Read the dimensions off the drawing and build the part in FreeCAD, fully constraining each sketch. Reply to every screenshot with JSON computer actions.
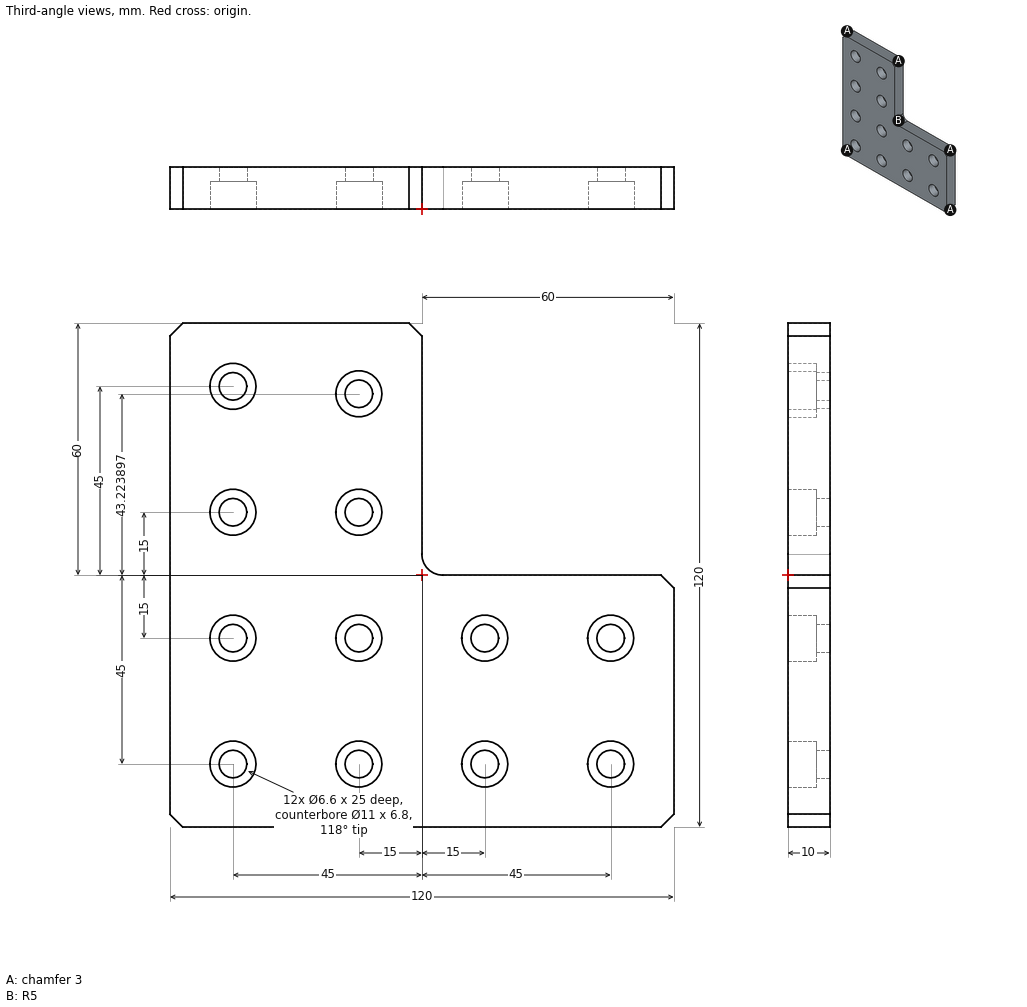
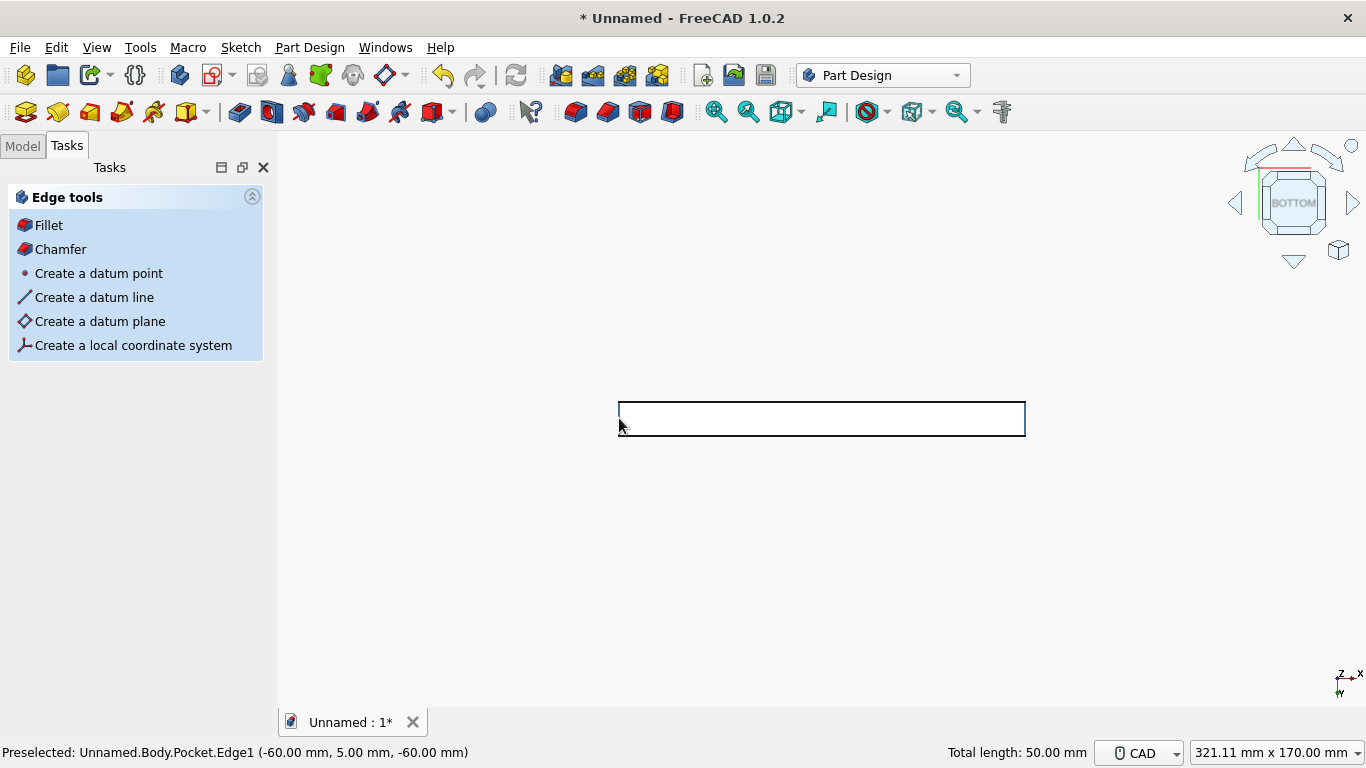
{"action": "left_click", "coordinate": [608, 112]}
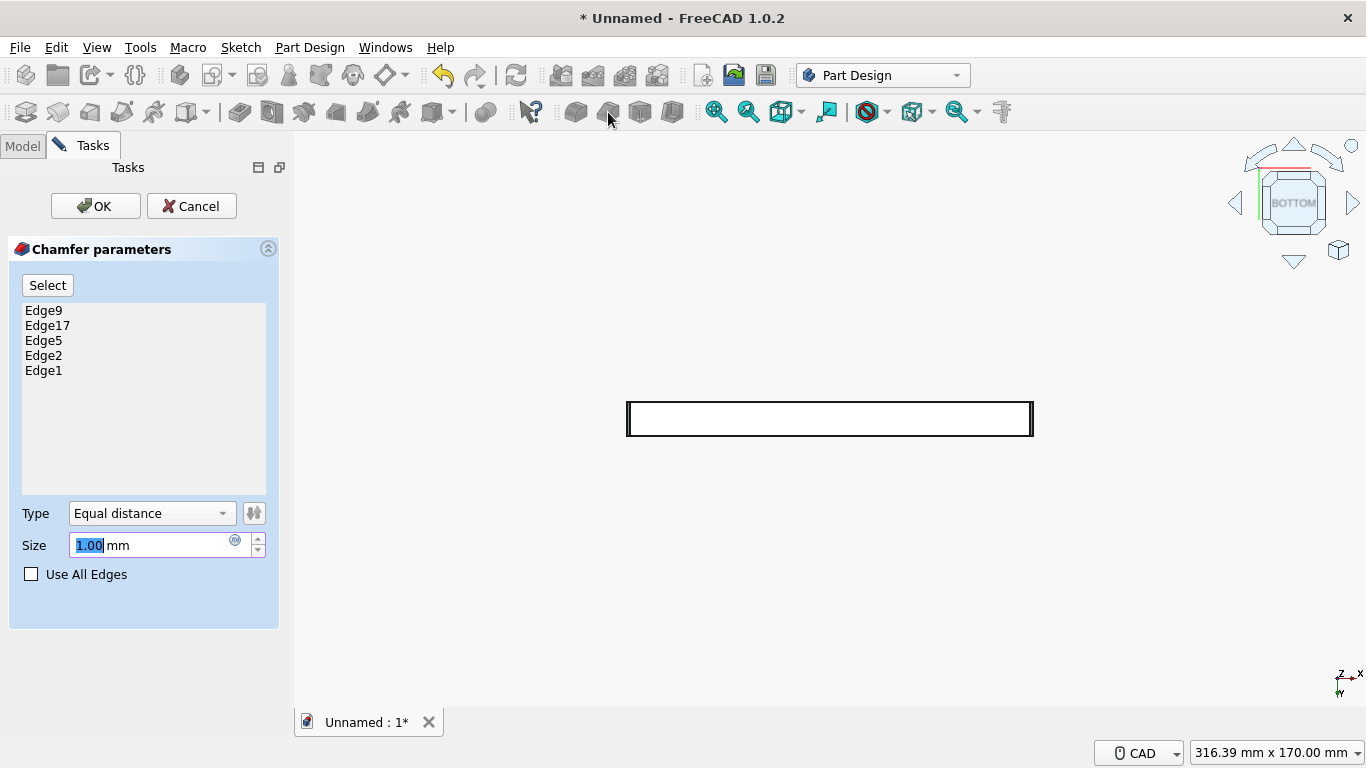
{"action": "type", "text": "3"}
{"action": "key", "text": "Tab"}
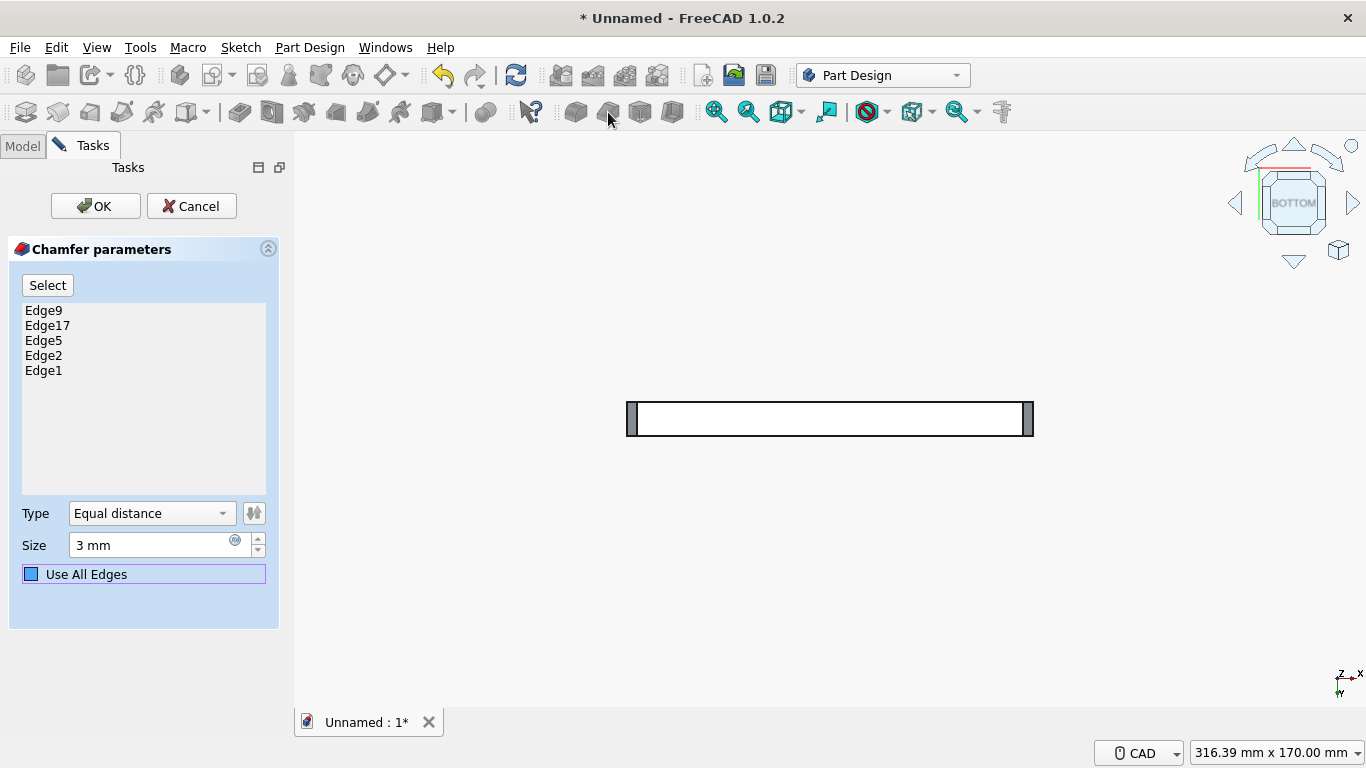
{"action": "left_click", "coordinate": [96, 206]}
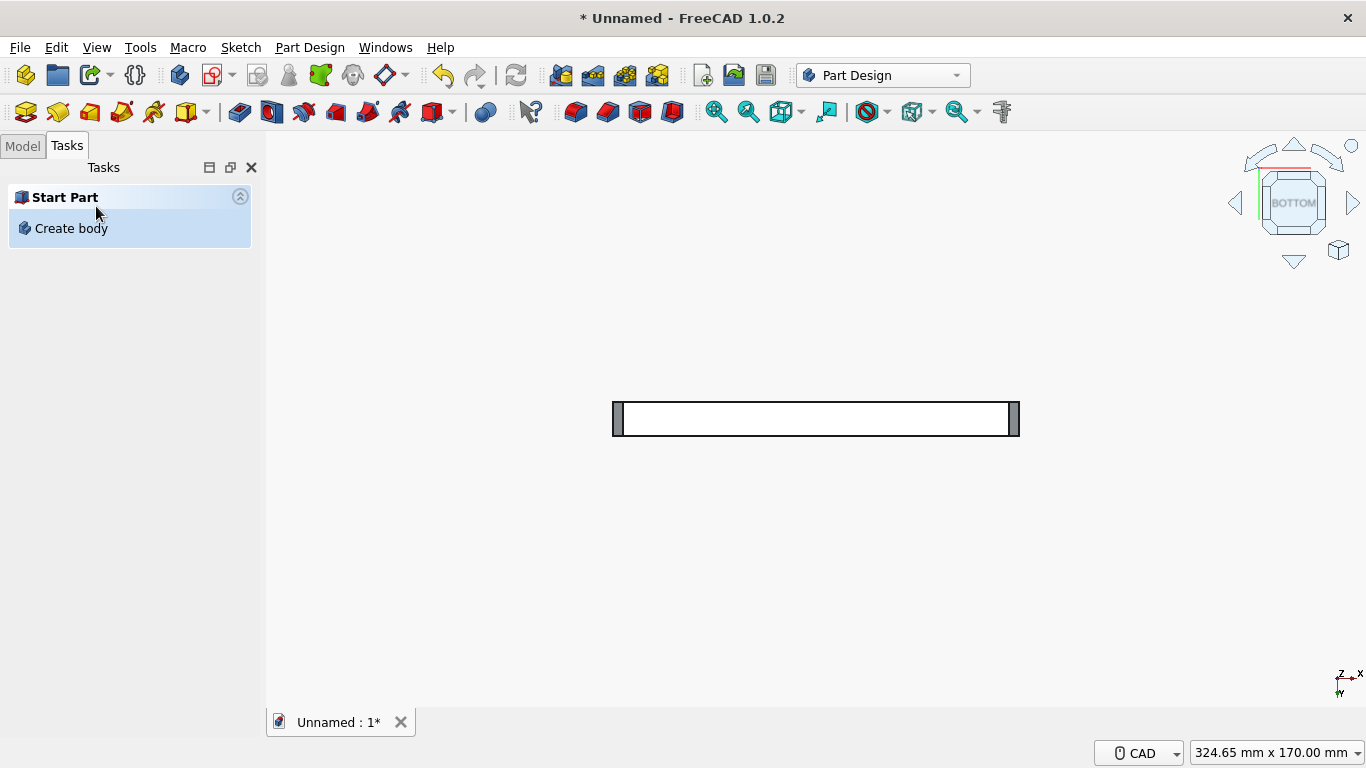
{"action": "left_click", "coordinate": [718, 112]}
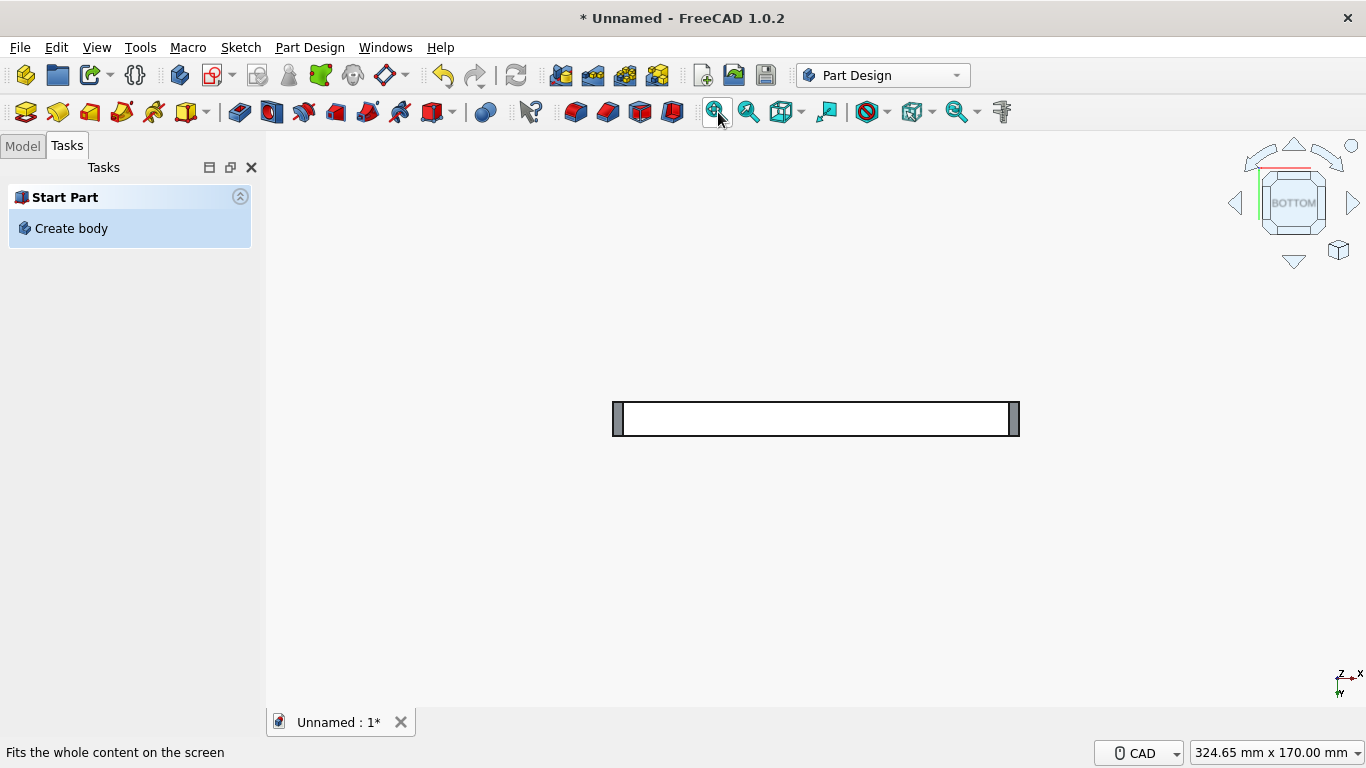
{"action": "key", "text": "0"}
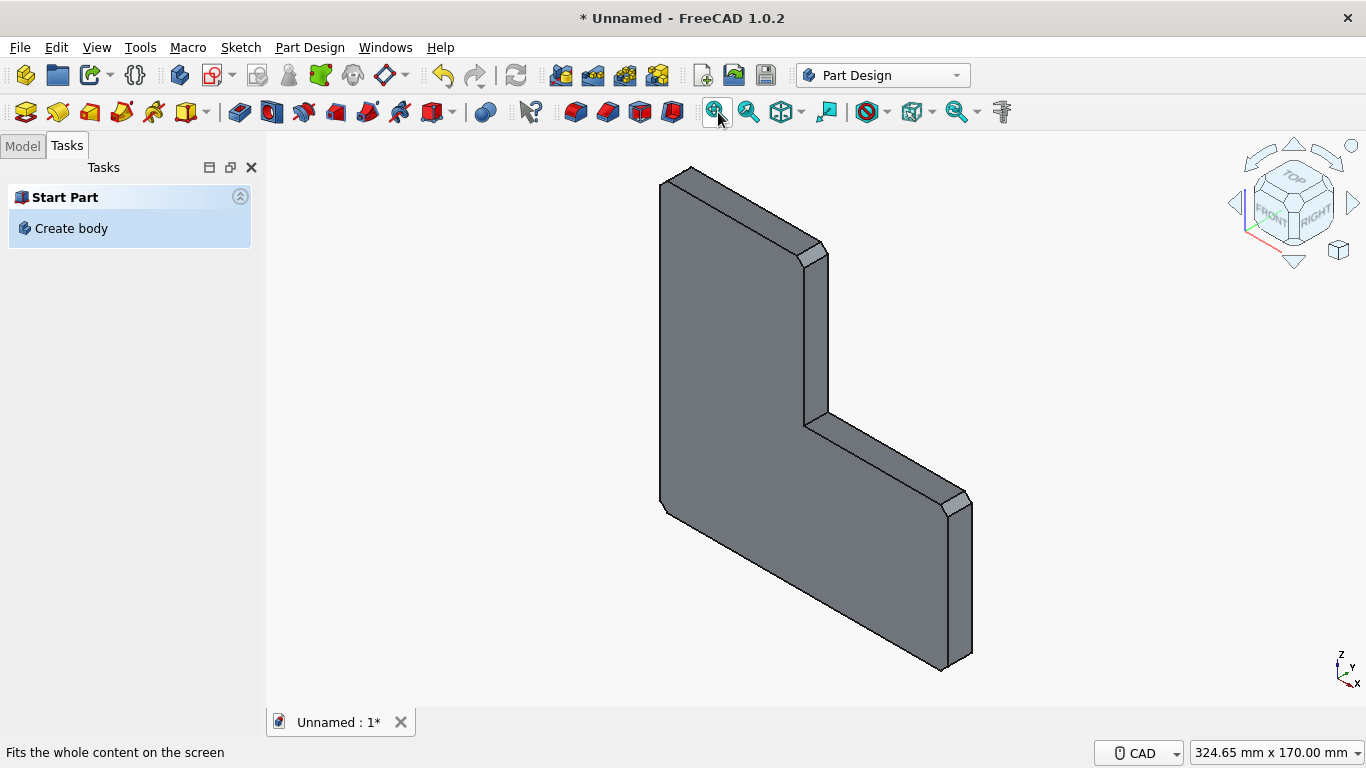
{"action": "key", "text": "2"}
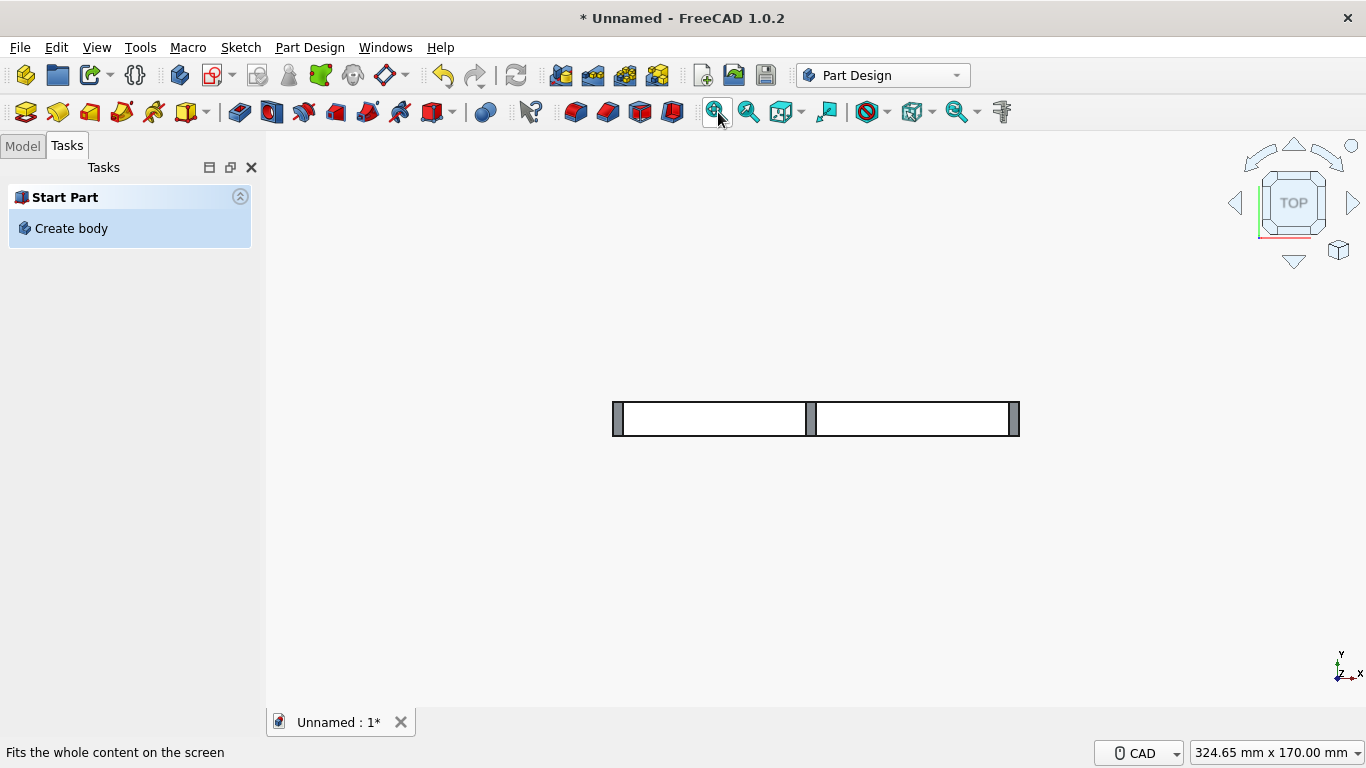
{"action": "left_click", "coordinate": [718, 112]}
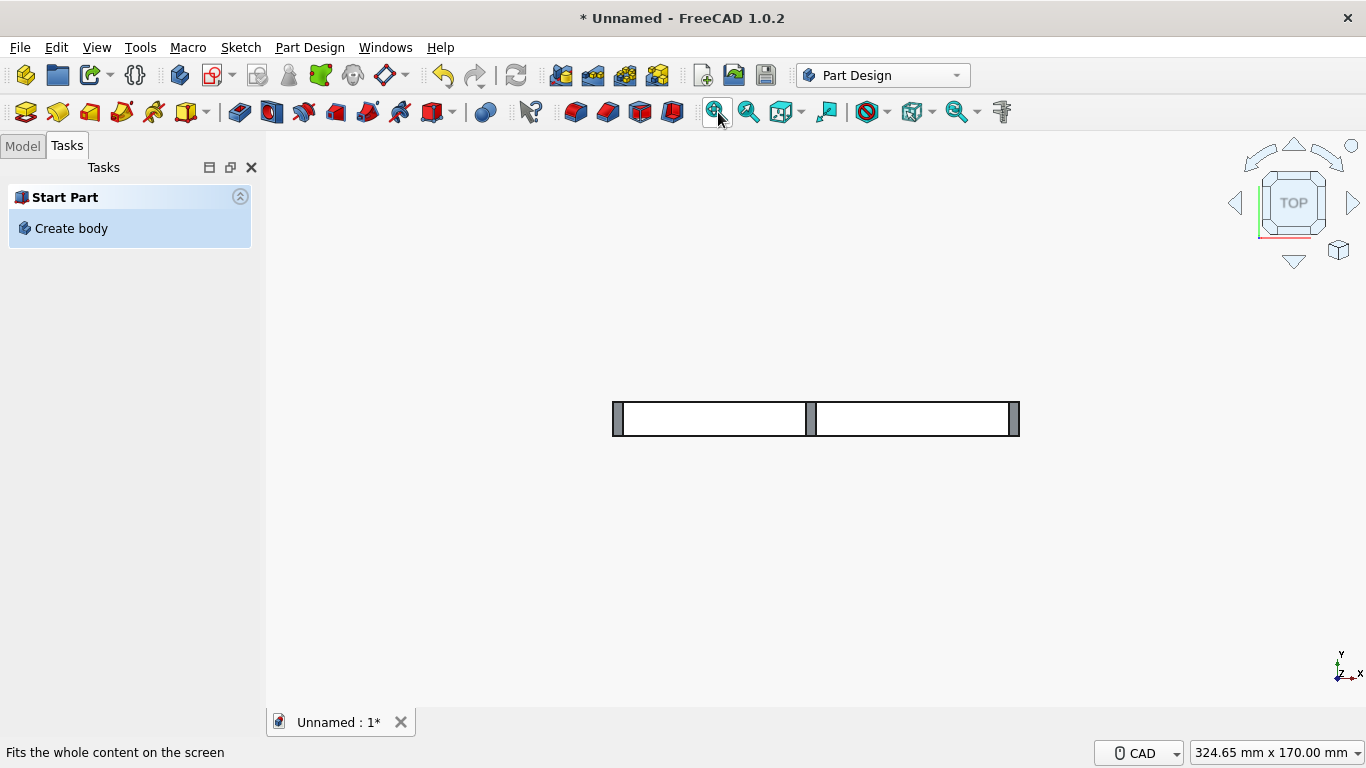
{"action": "key", "text": "1"}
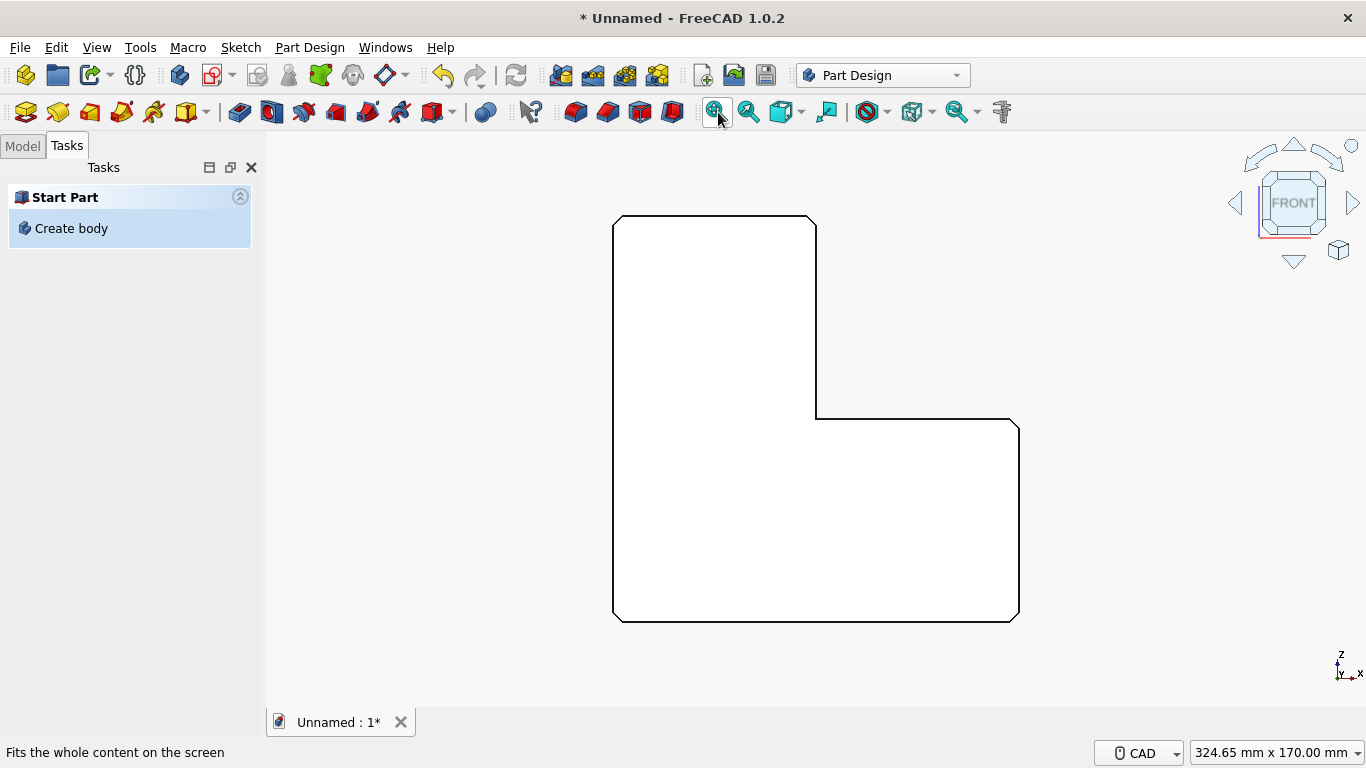
{"action": "key", "text": "3"}